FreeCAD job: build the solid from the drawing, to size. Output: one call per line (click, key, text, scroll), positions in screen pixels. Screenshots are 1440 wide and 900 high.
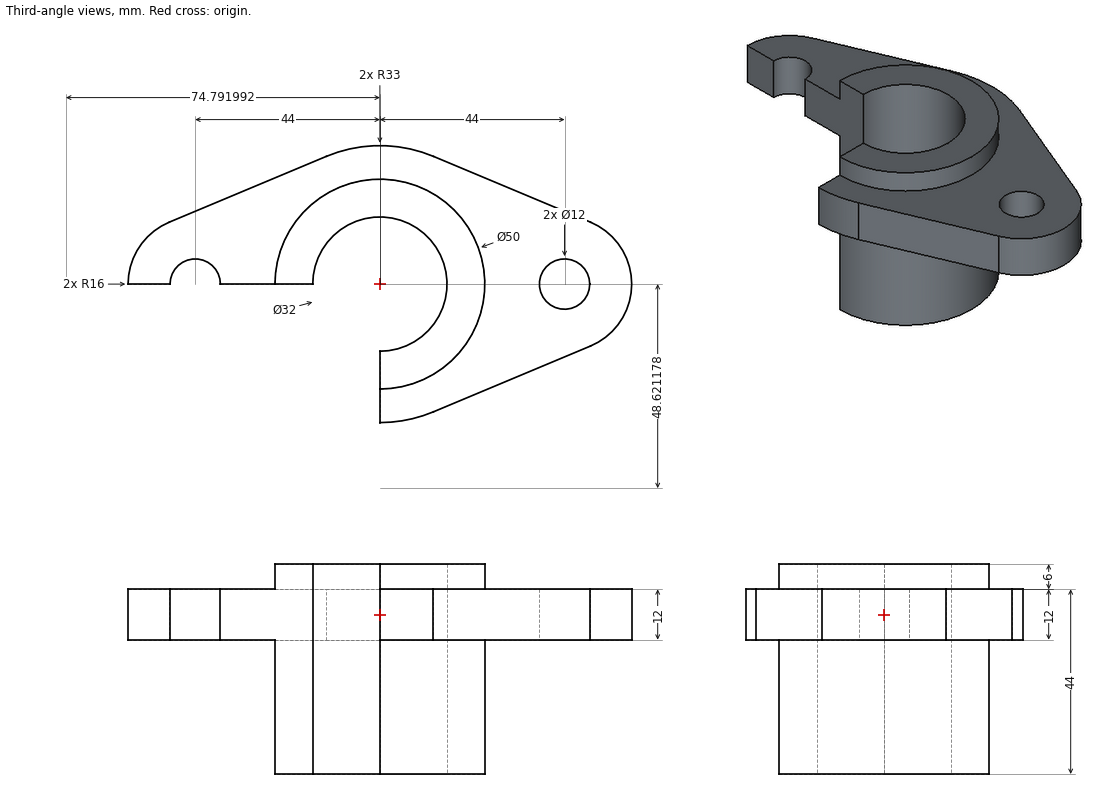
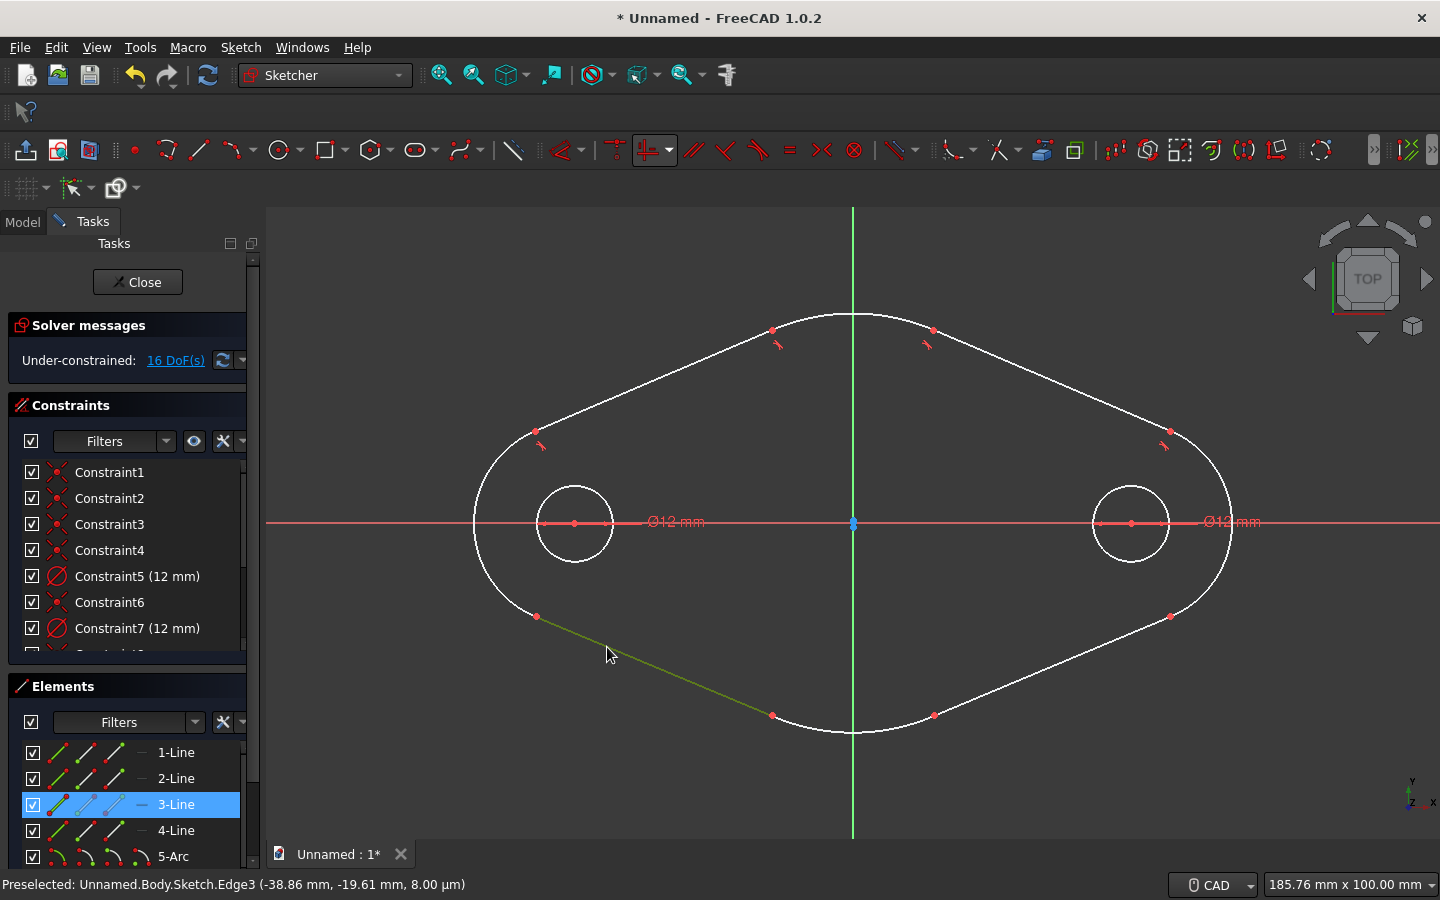
click(485, 479)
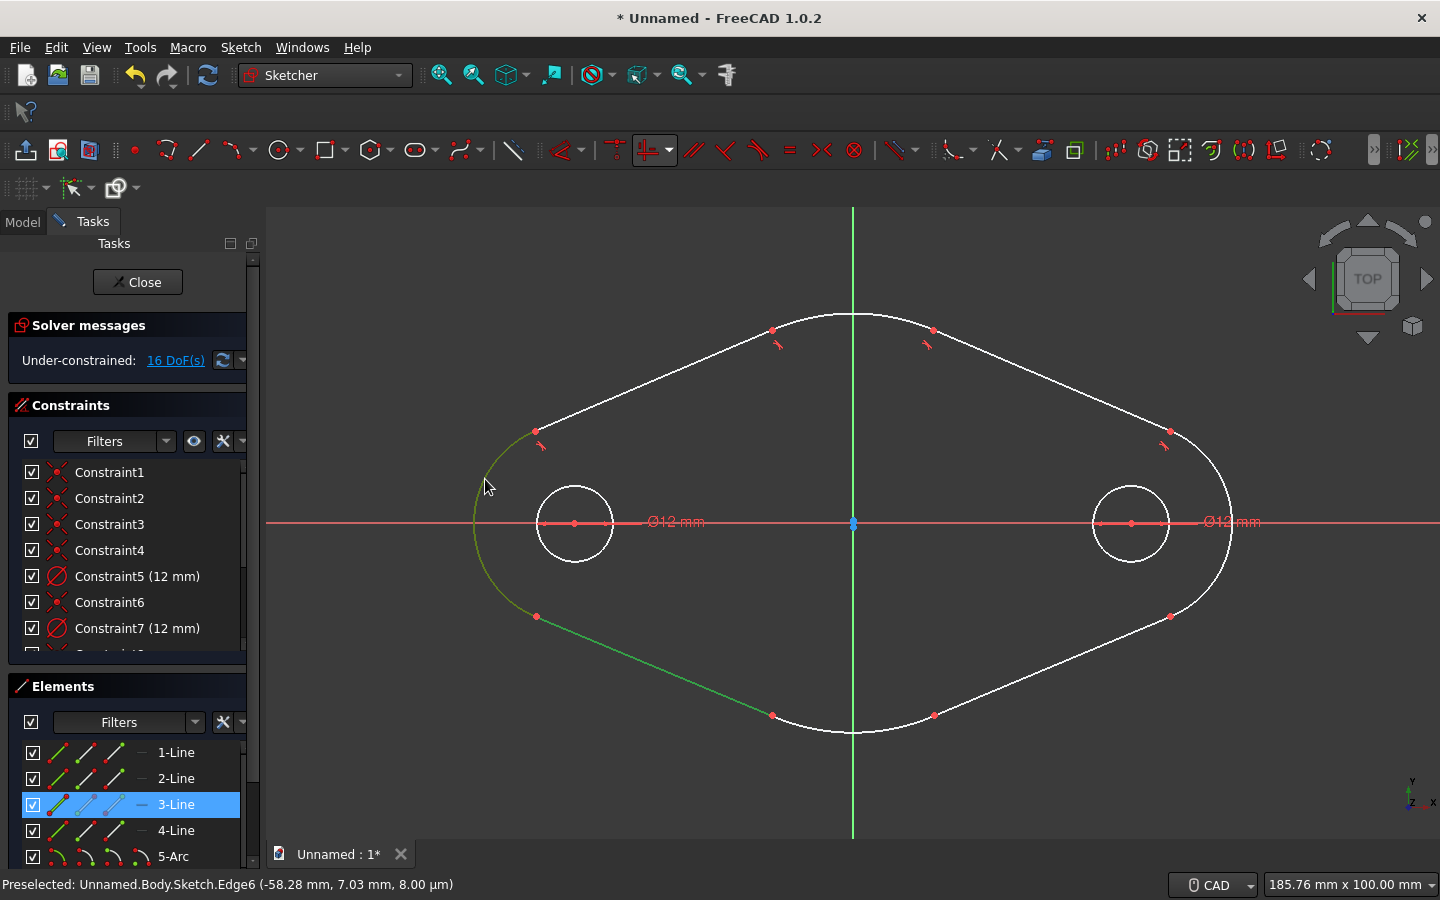
click(758, 150)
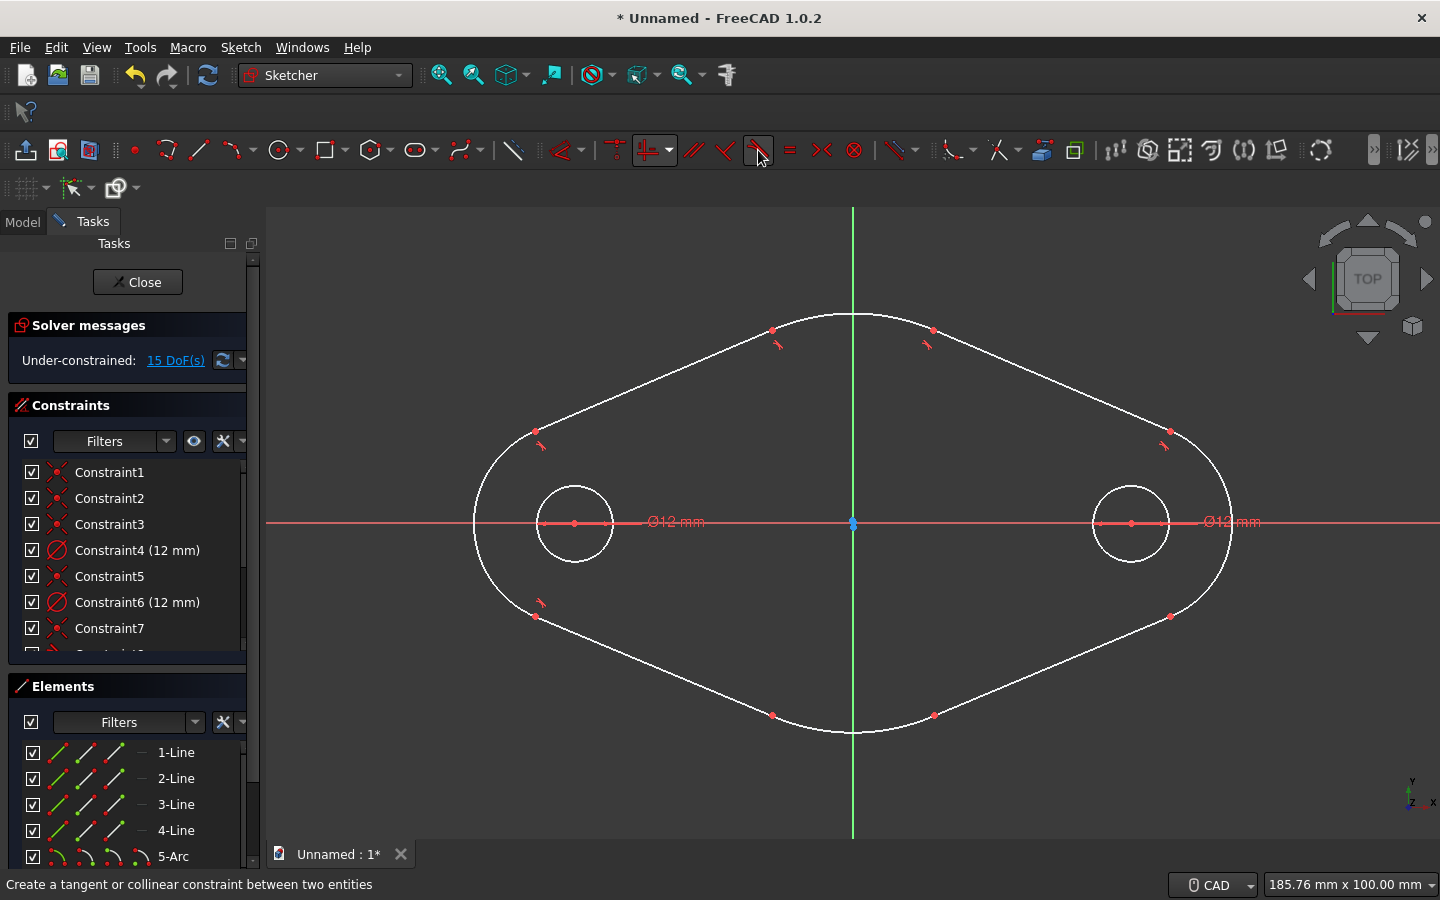
click(607, 647)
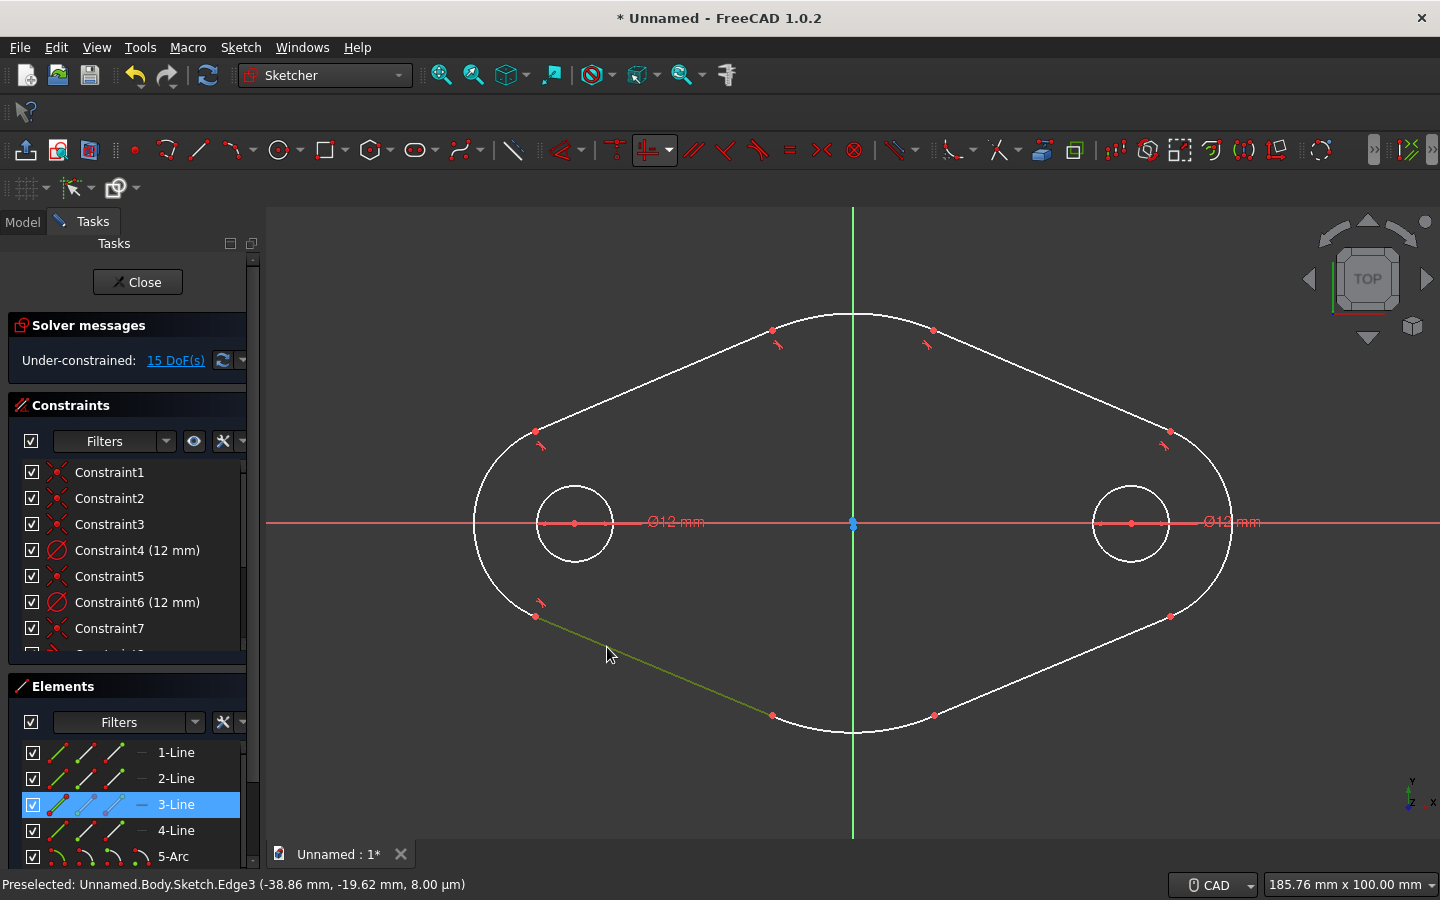
click(820, 730)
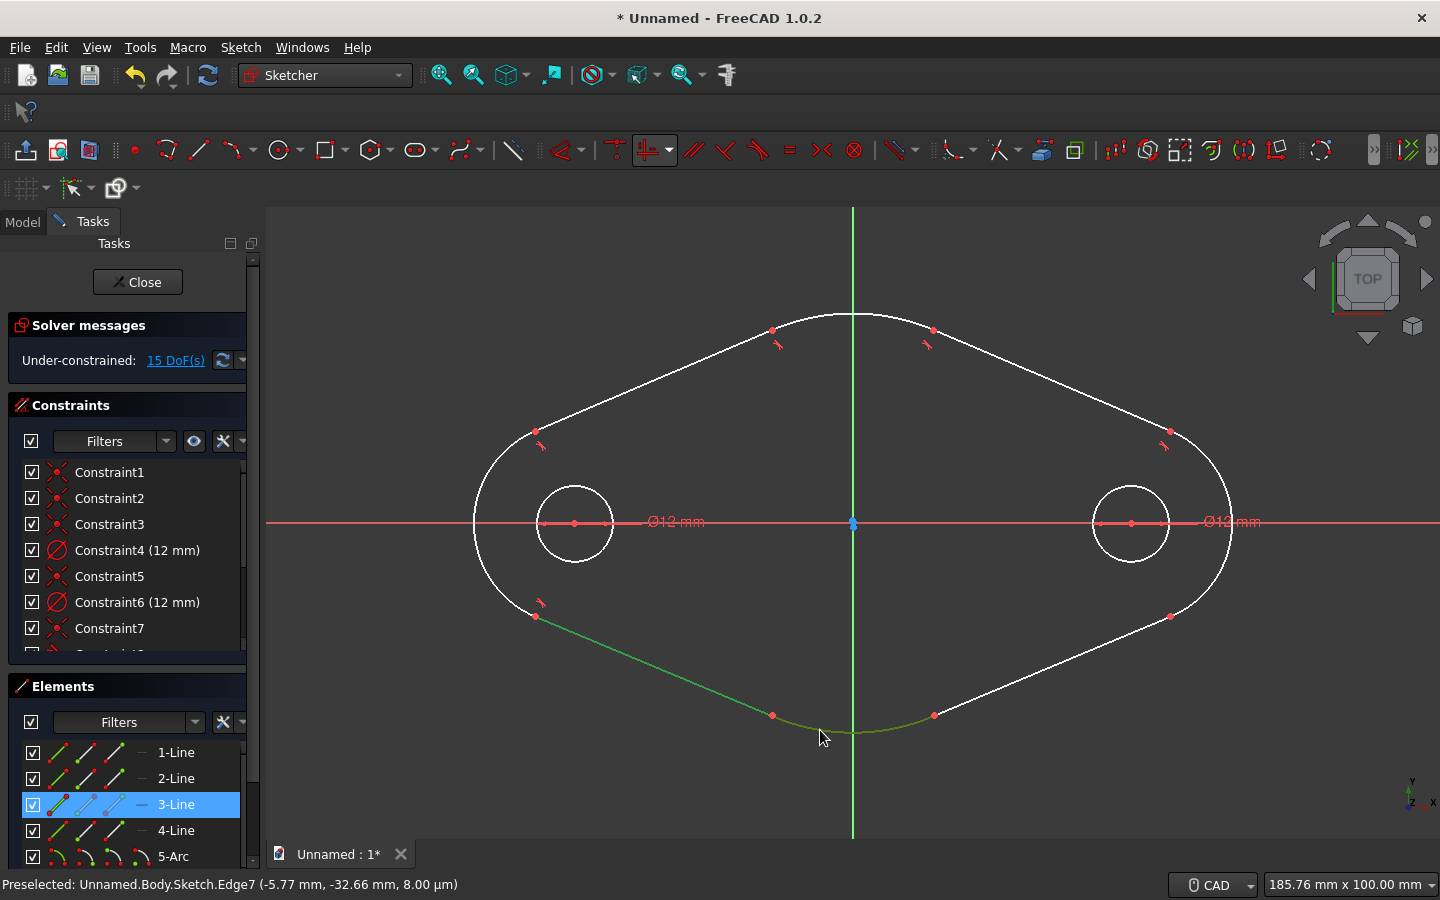
click(758, 150)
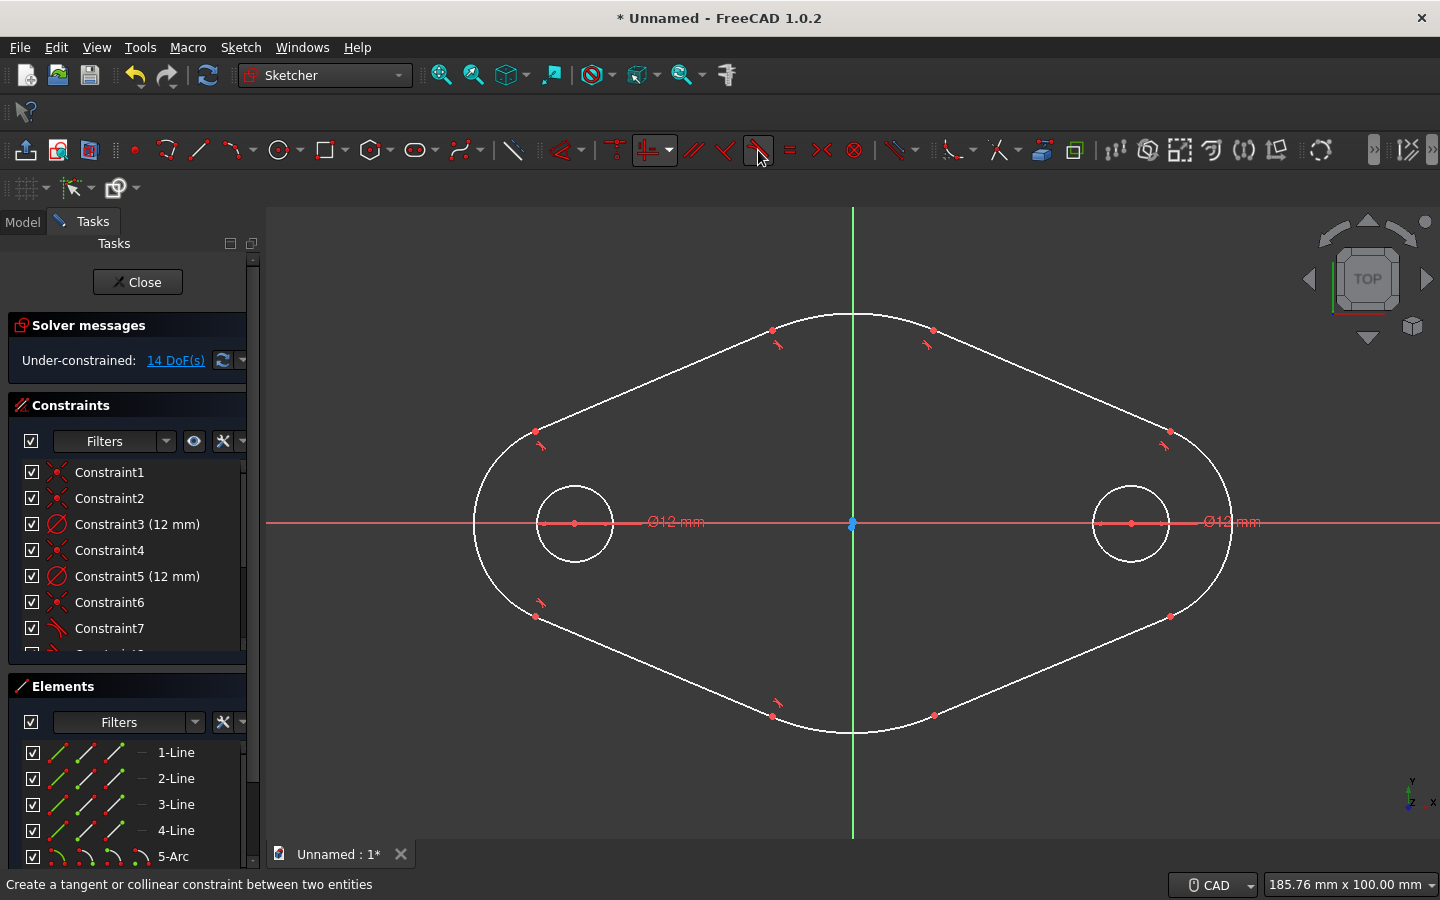
click(1005, 686)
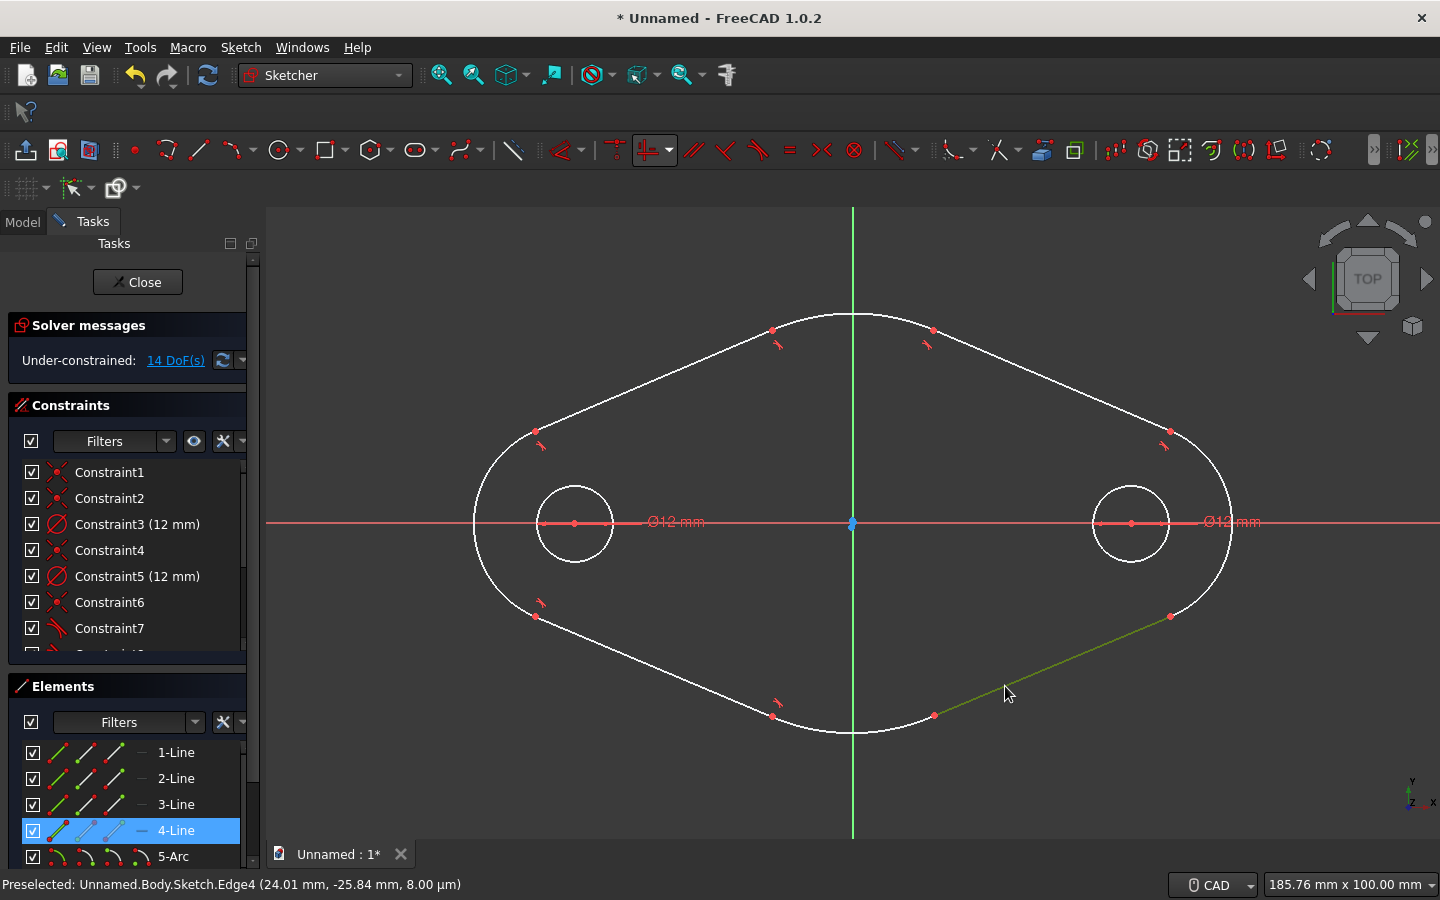
click(820, 731)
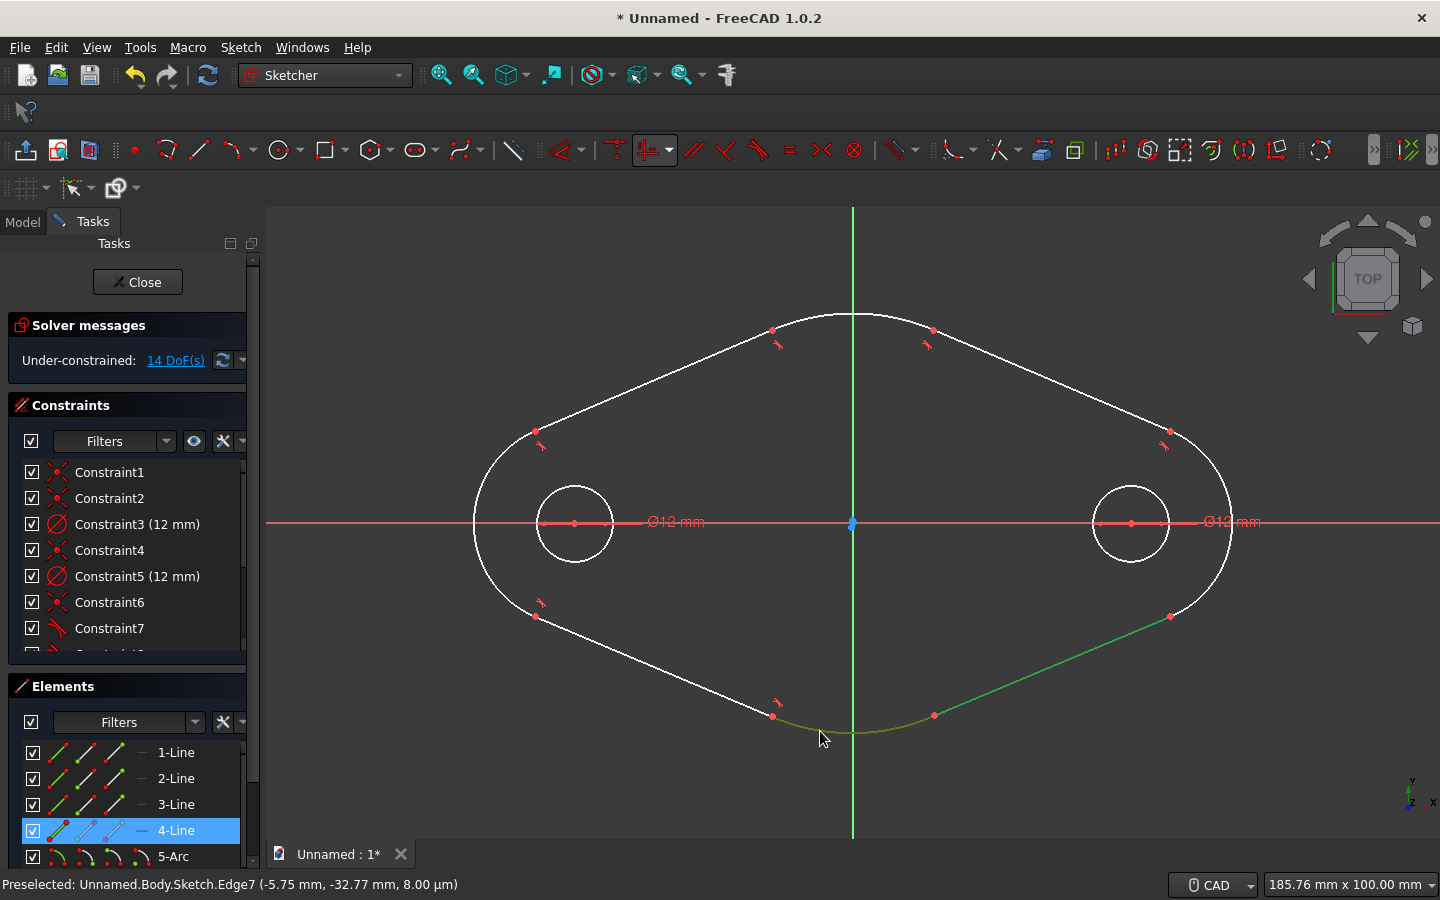
click(758, 150)